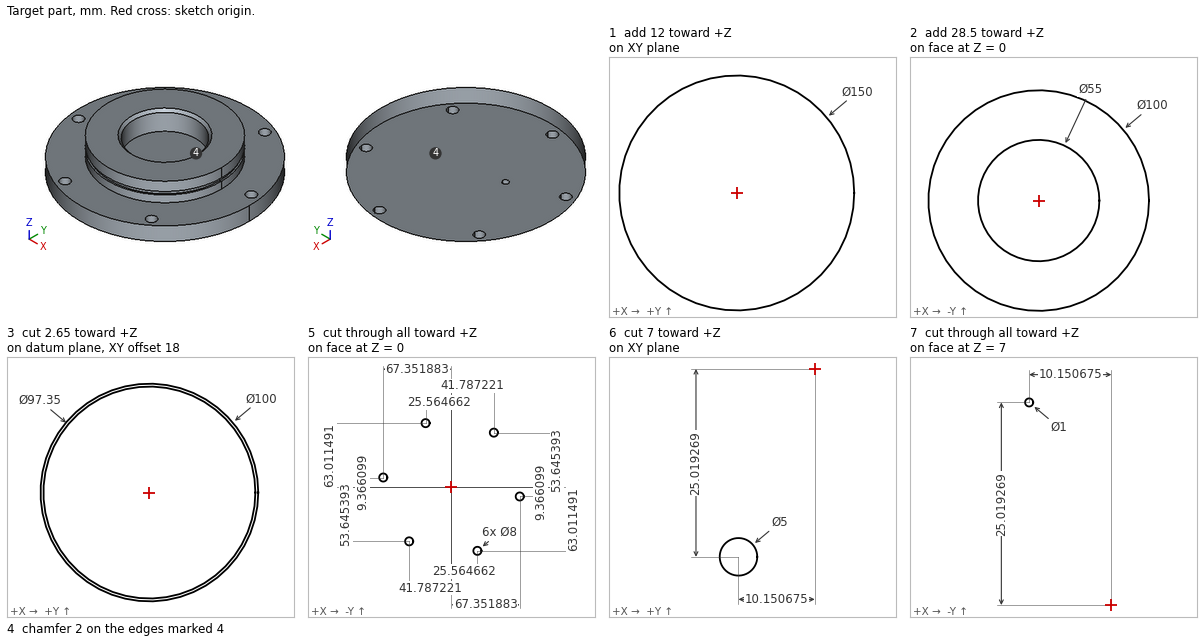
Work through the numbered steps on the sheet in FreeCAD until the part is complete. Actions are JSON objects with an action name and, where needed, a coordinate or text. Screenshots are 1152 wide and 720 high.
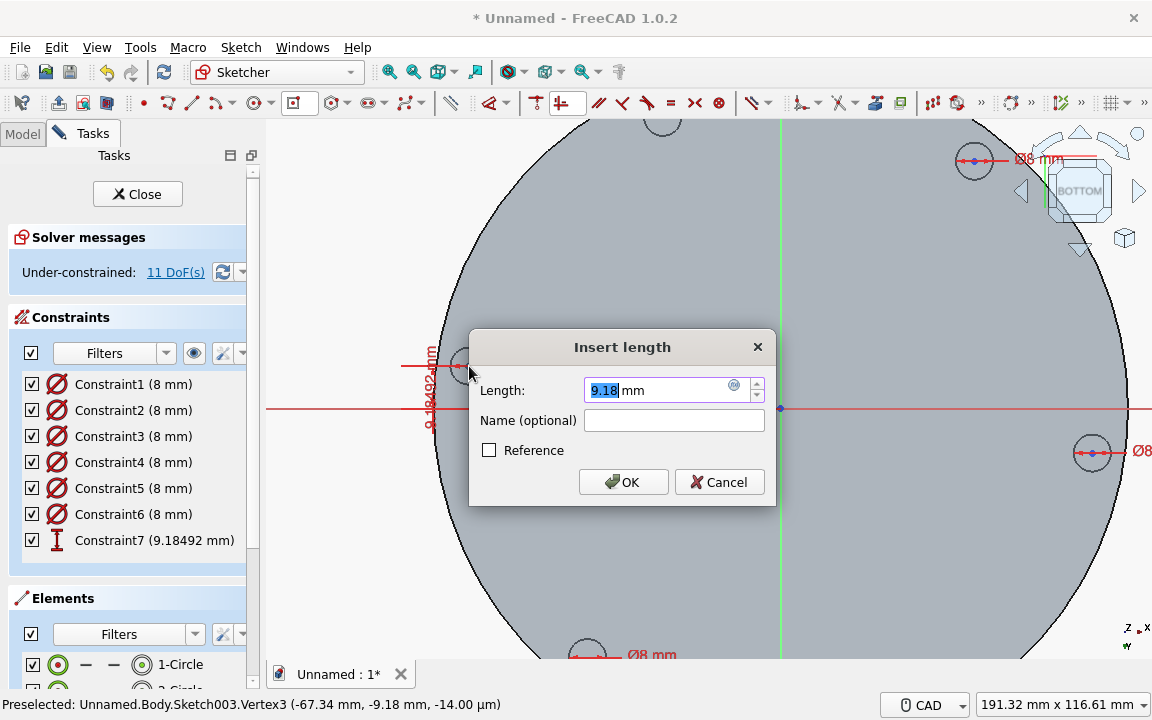
{"action": "type", "text": "9.366099"}
{"action": "key", "text": "Return"}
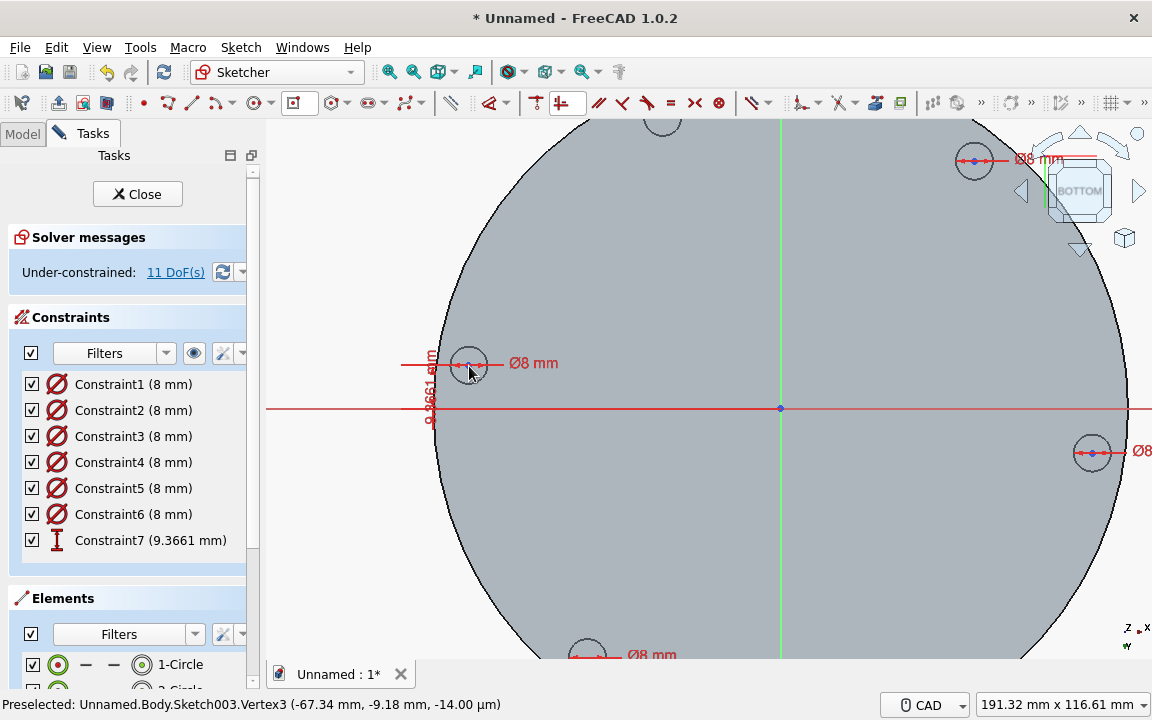
{"action": "scroll", "coordinate": [470, 365], "scroll_direction": "down", "scroll_amount": 3}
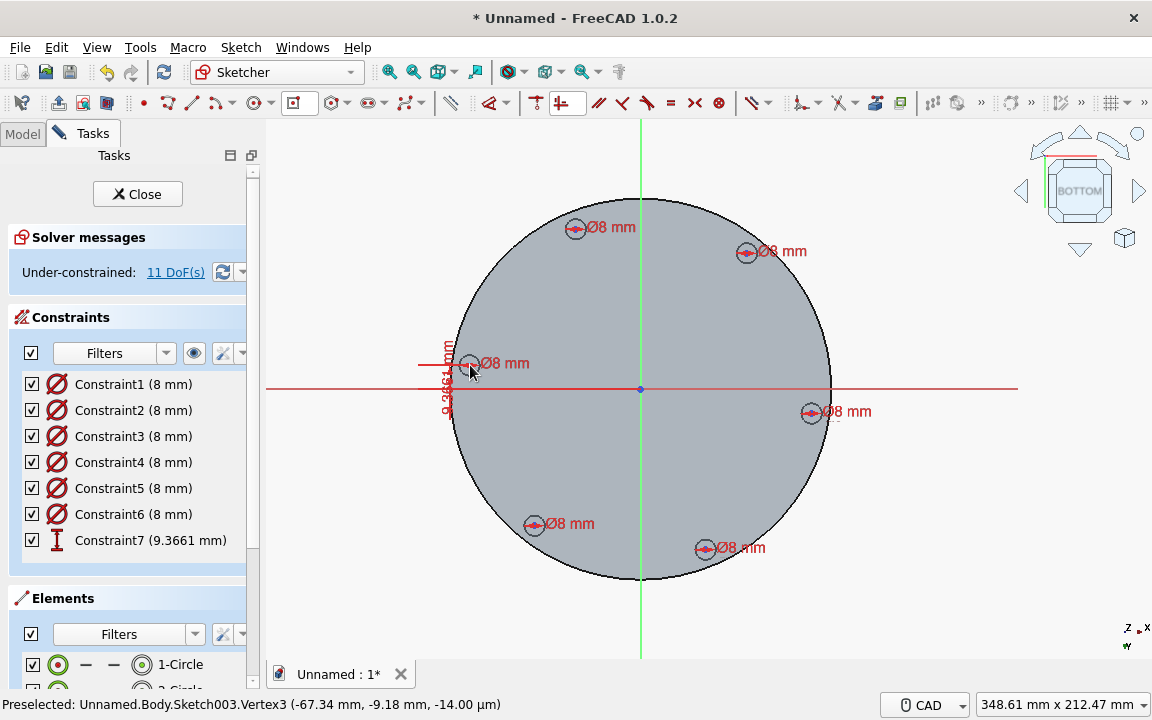
{"action": "scroll", "coordinate": [812, 414], "scroll_direction": "up", "scroll_amount": 3}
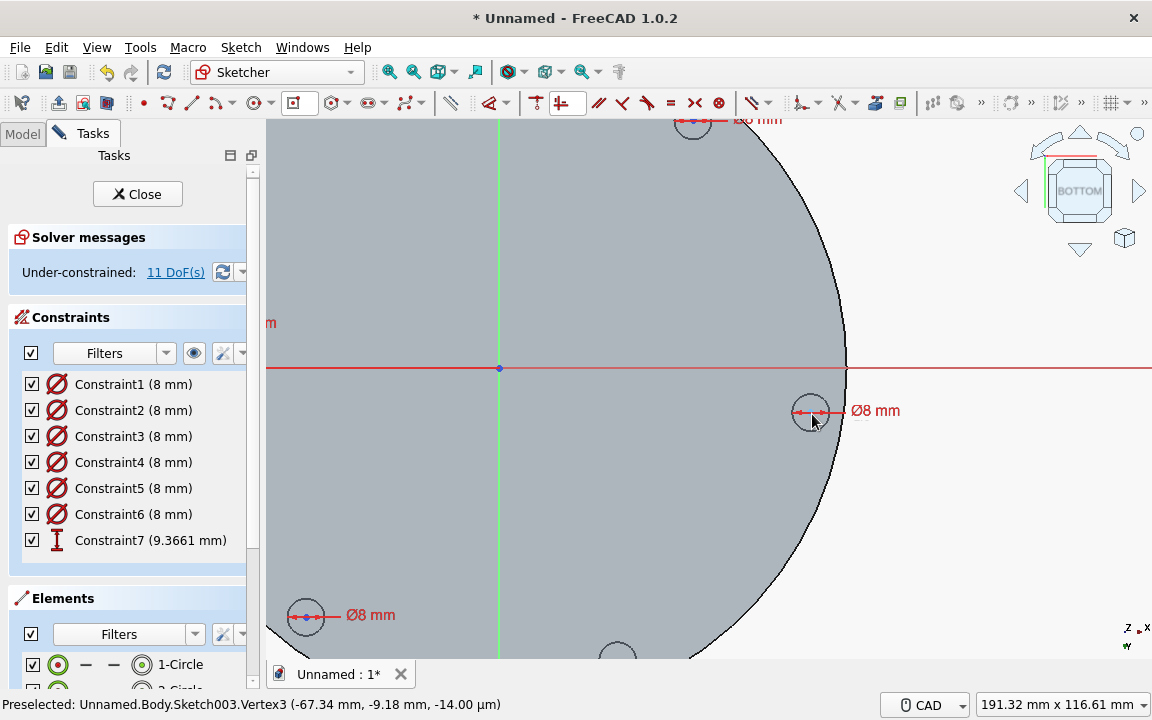
{"action": "left_click", "coordinate": [811, 413]}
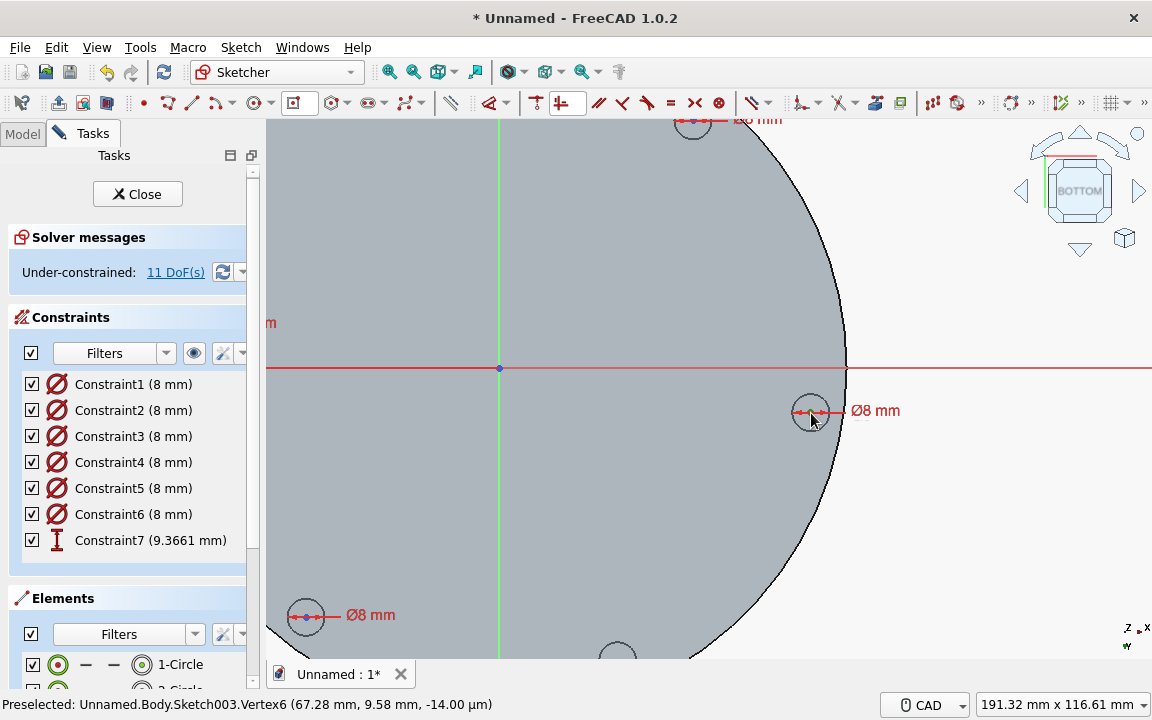
{"action": "key", "text": "i"}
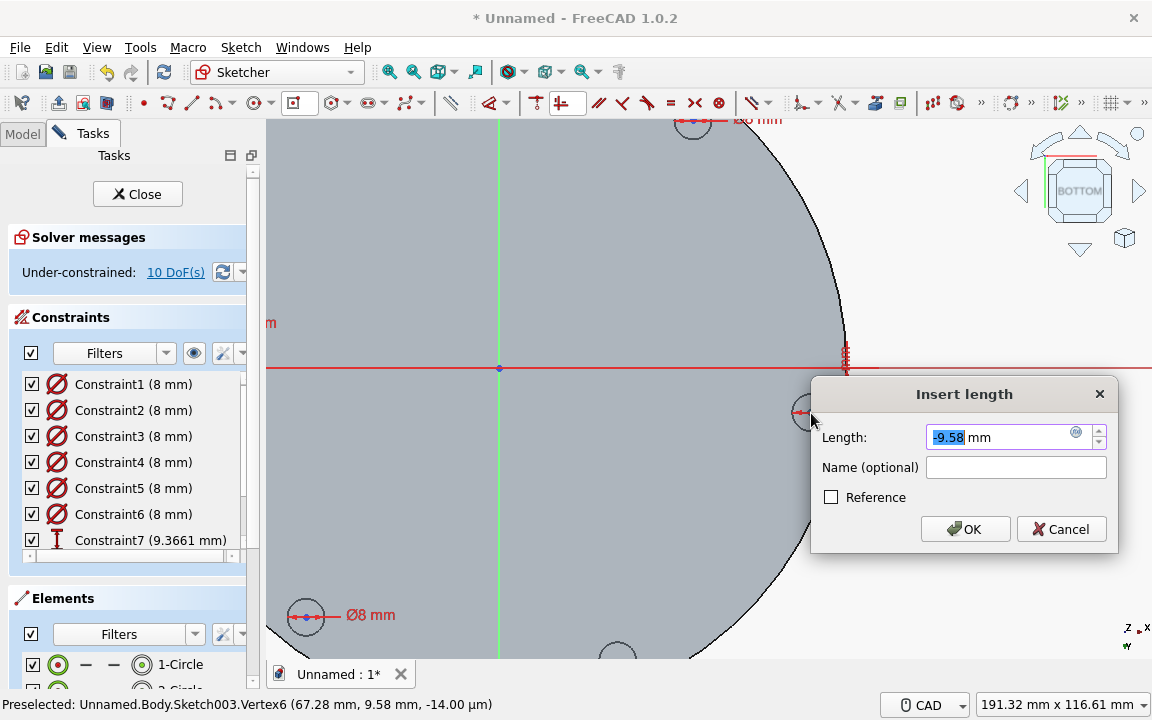
{"action": "type", "text": "-9.366099"}
{"action": "key", "text": "Return"}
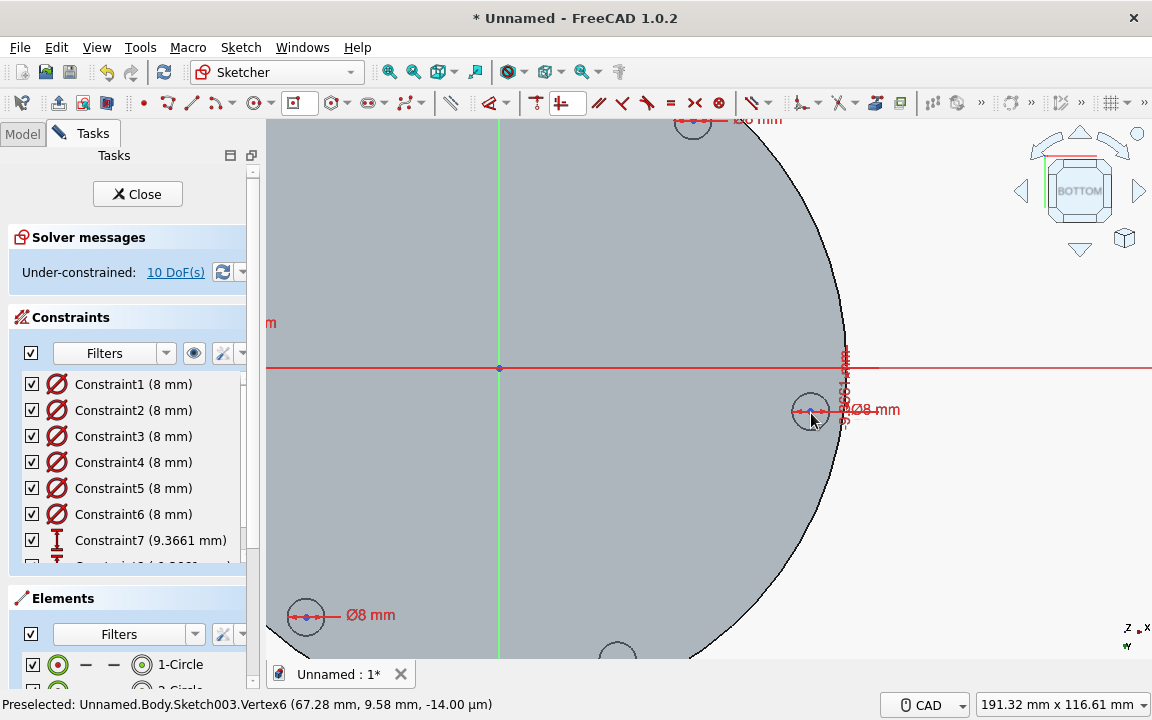
{"action": "scroll", "coordinate": [812, 414], "scroll_direction": "down", "scroll_amount": 3}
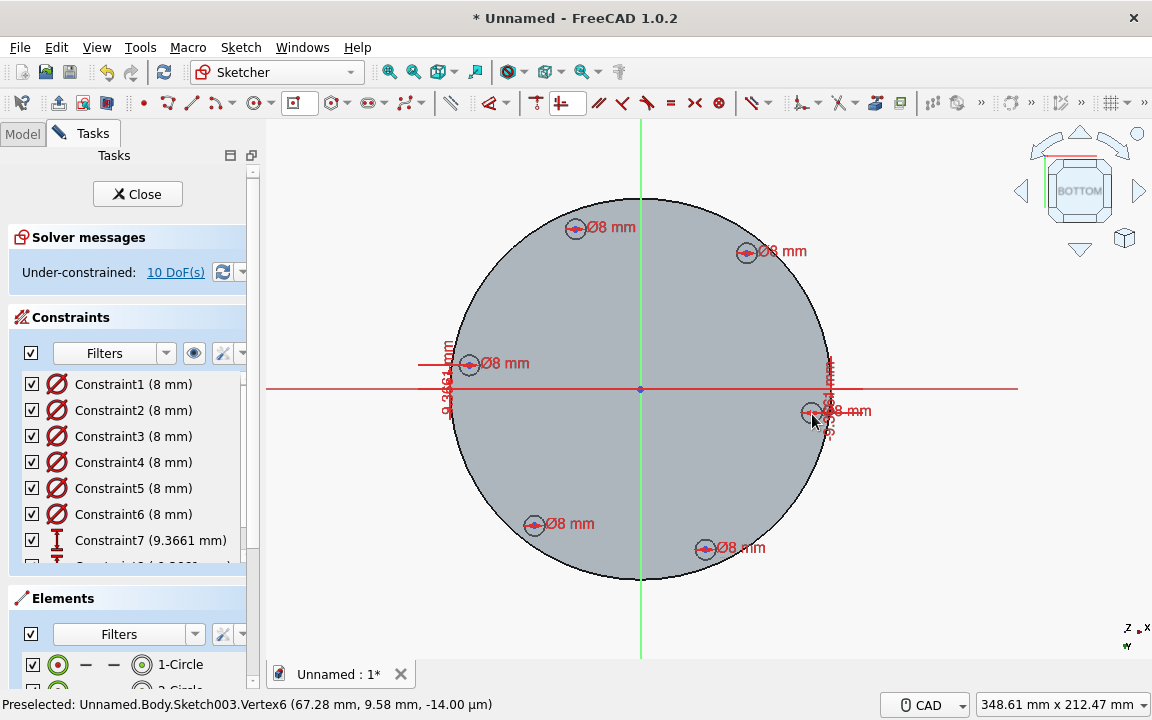
{"action": "left_click", "coordinate": [706, 550]}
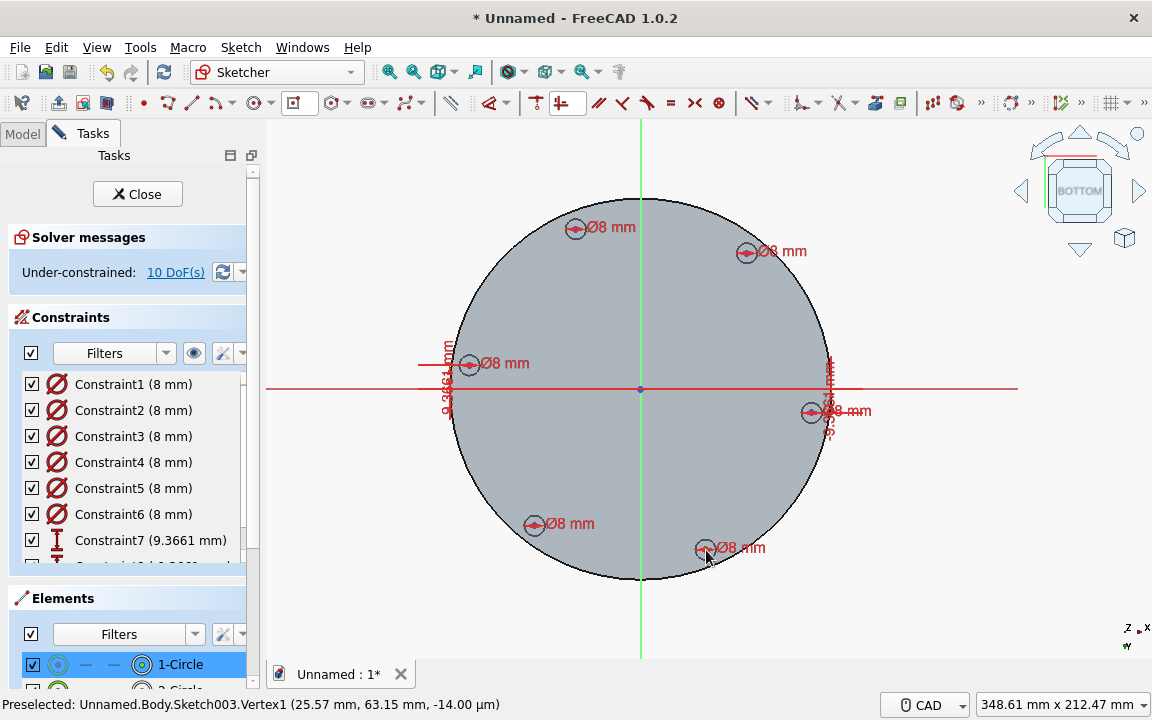
{"action": "key", "text": "l"}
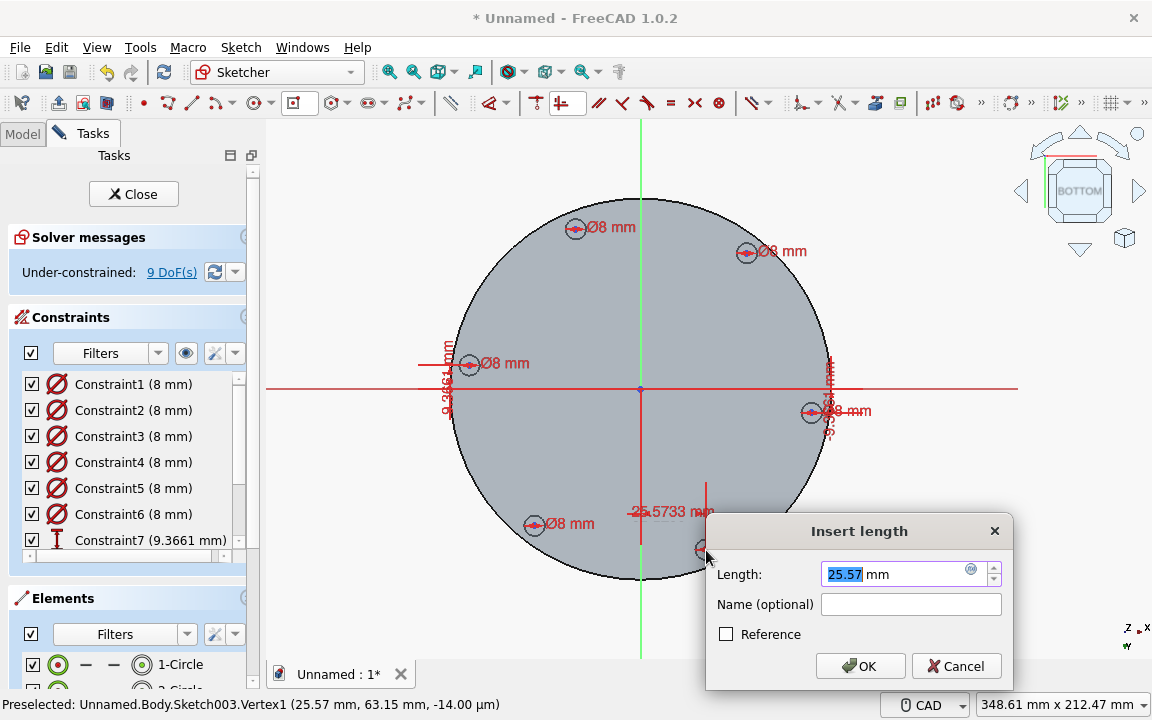
{"action": "type", "text": "25.564662"}
{"action": "key", "text": "Return"}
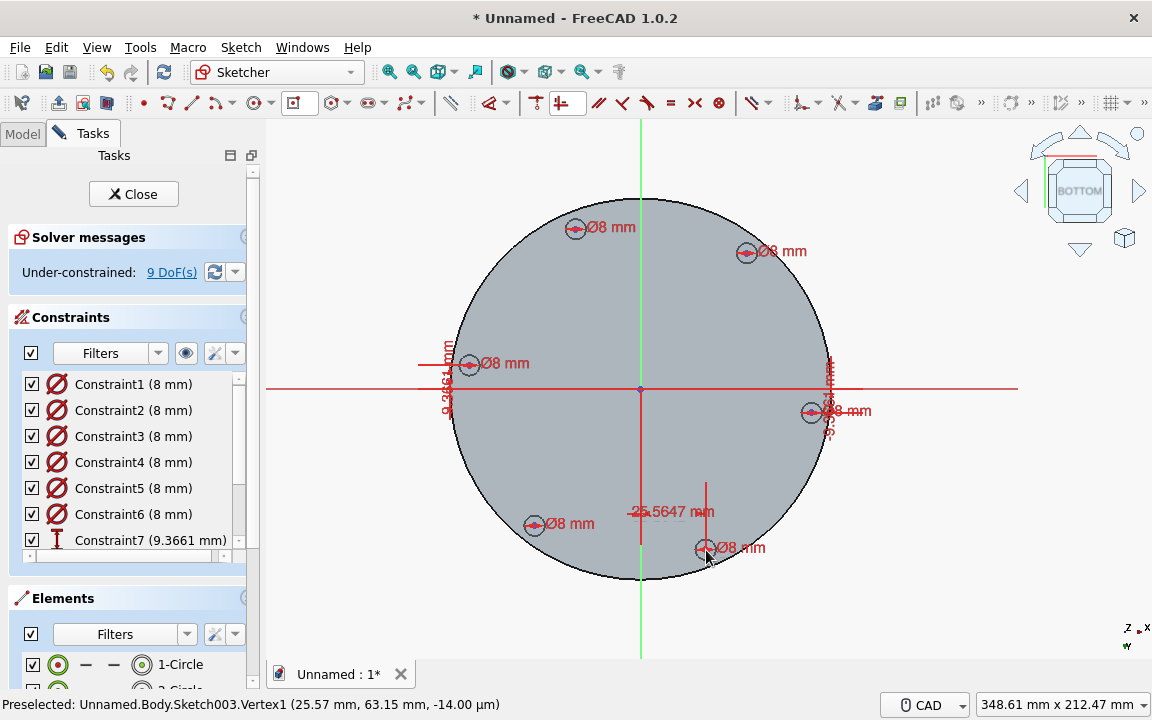
{"action": "left_click", "coordinate": [706, 550]}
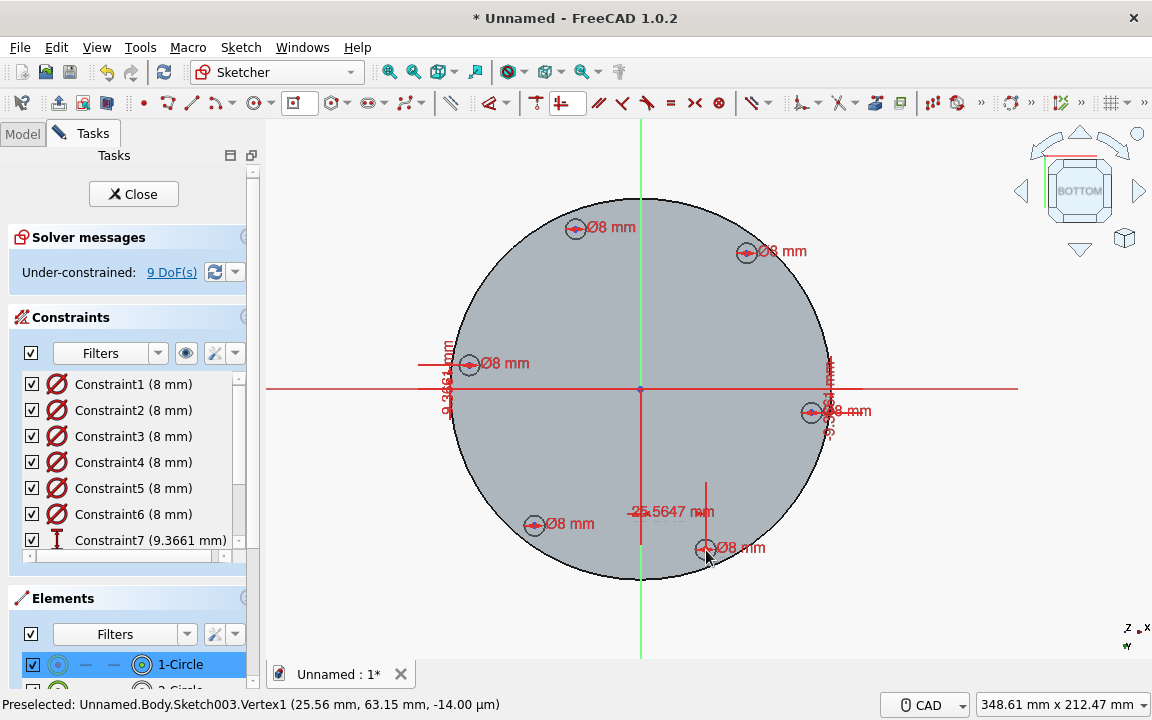
{"action": "key", "text": "i"}